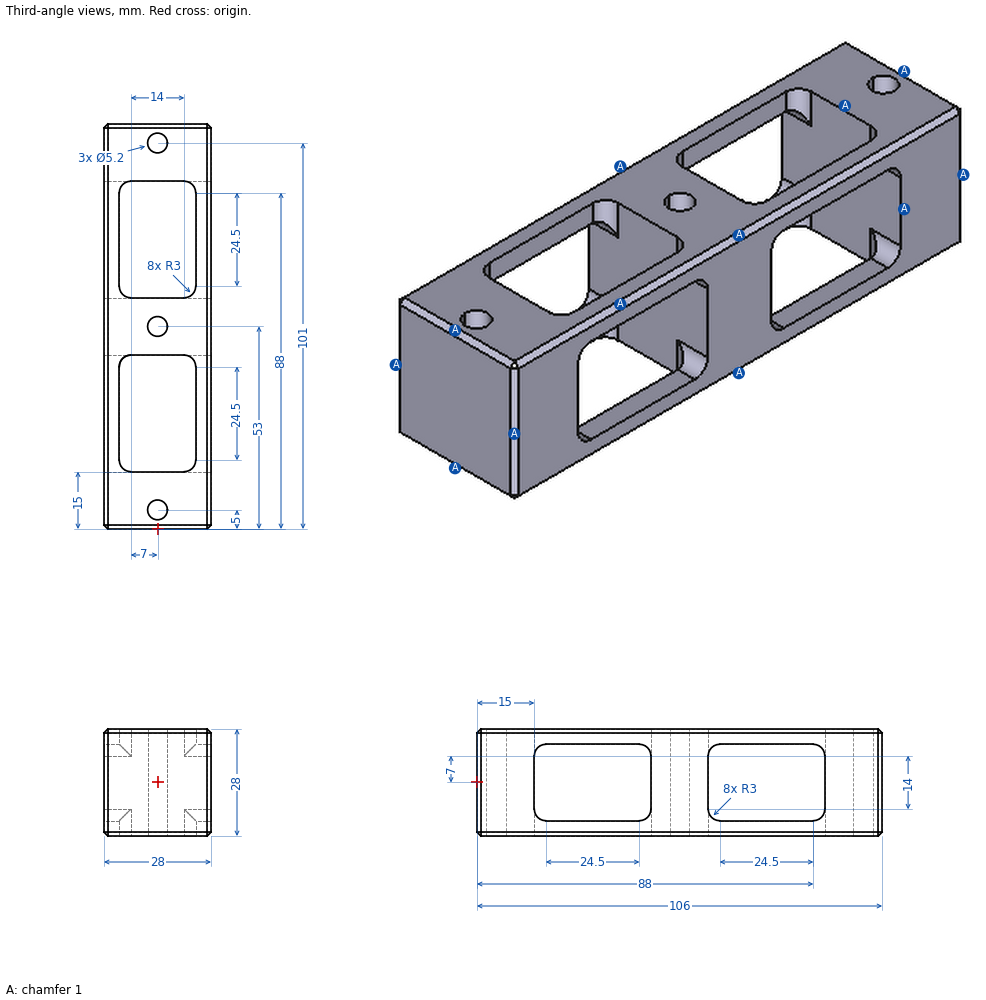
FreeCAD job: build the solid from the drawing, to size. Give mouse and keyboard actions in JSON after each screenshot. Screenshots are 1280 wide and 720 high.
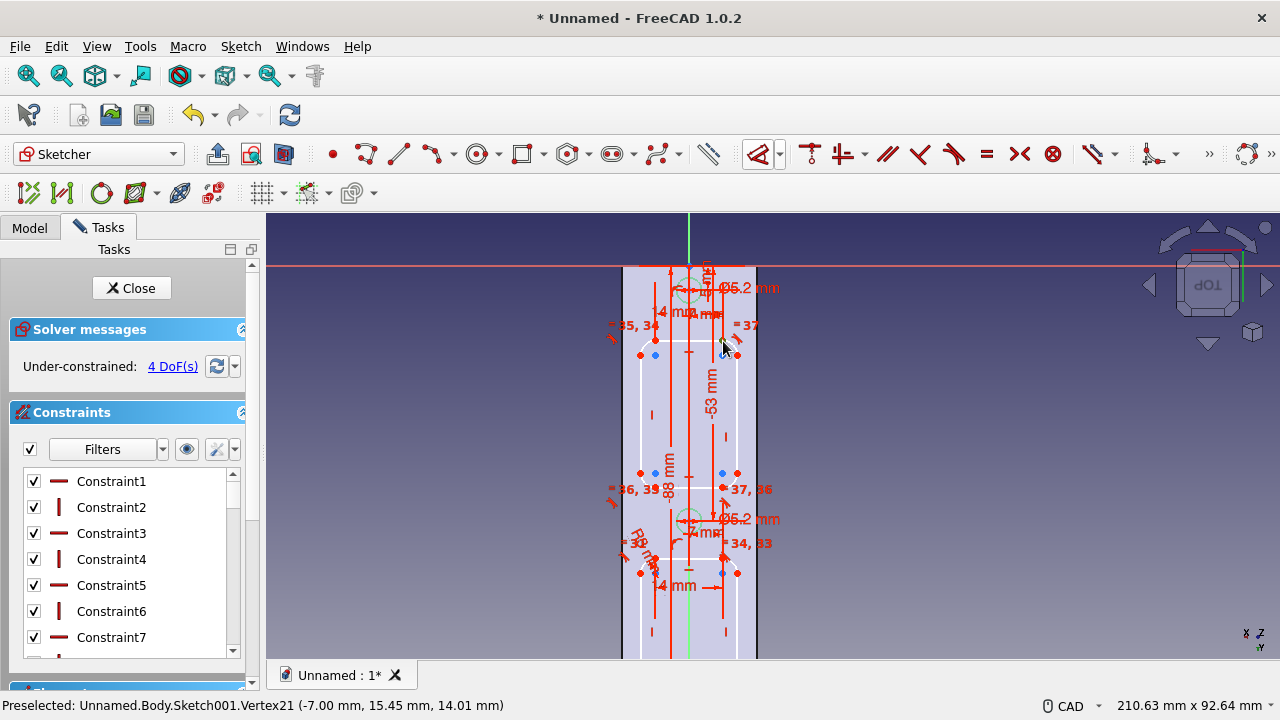
{"action": "key", "text": "i"}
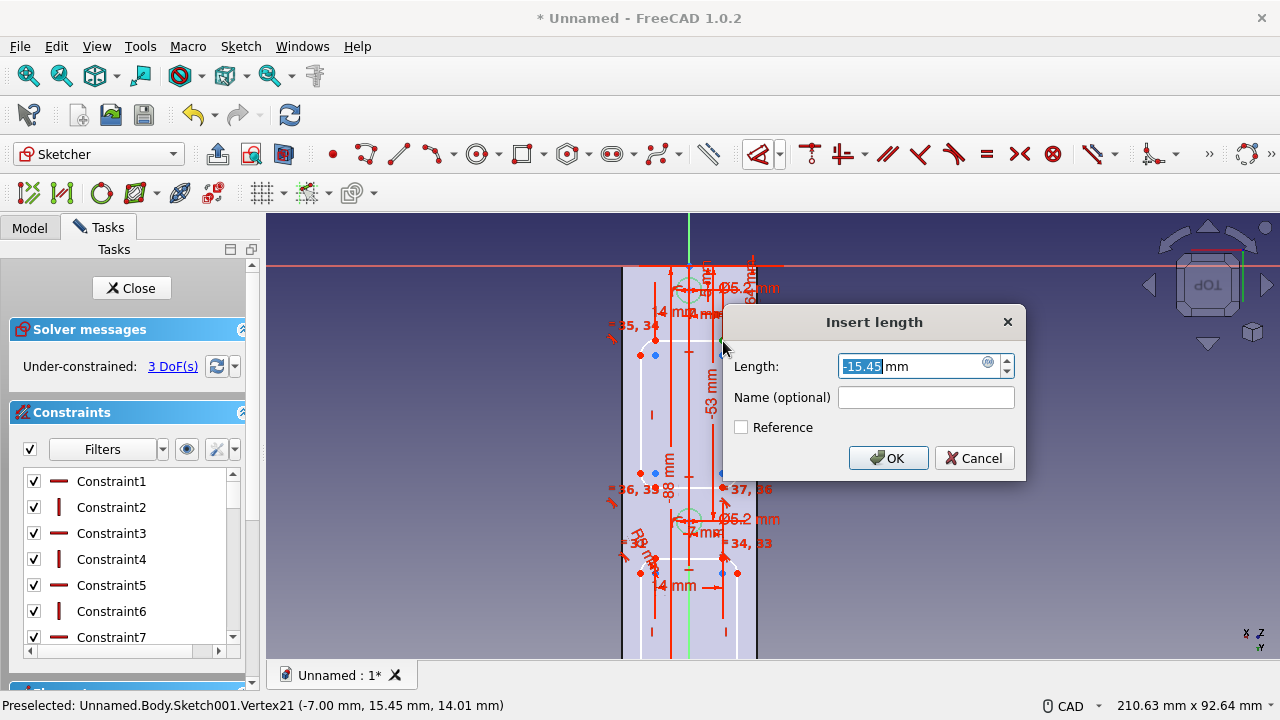
{"action": "type", "text": "-15"}
{"action": "key", "text": "Return"}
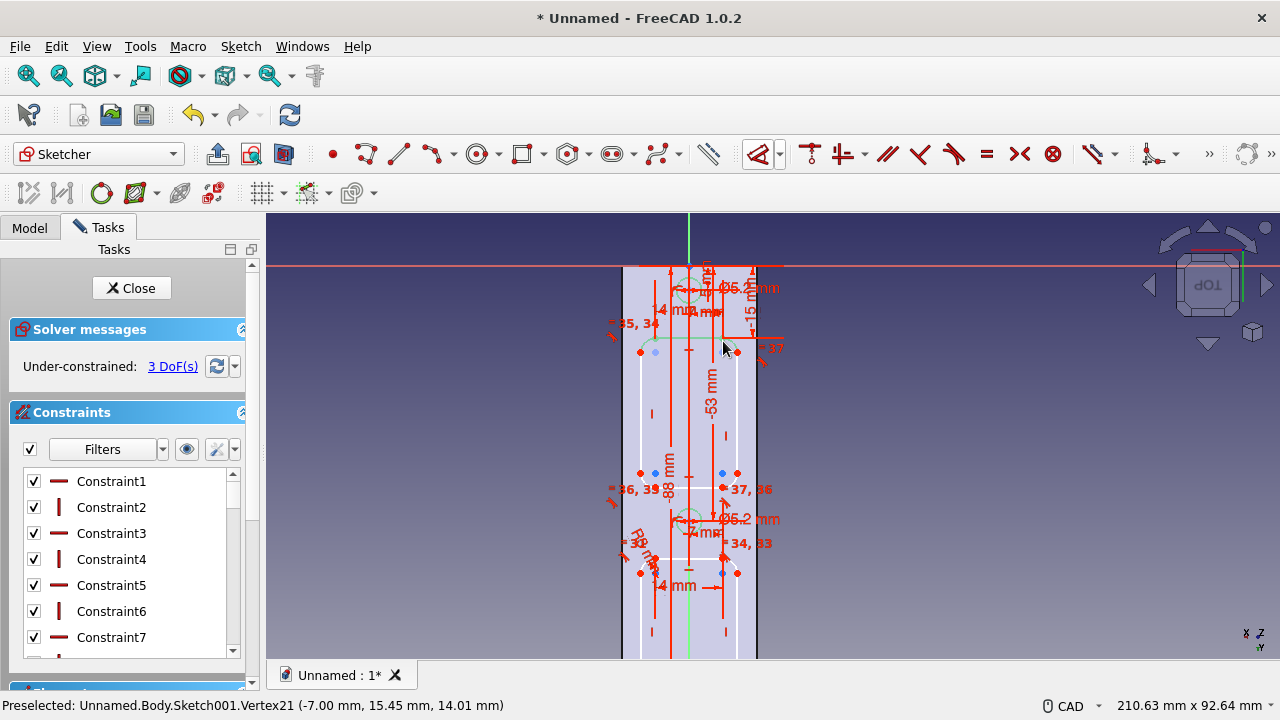
{"action": "scroll", "coordinate": [723, 339], "scroll_direction": "down", "scroll_amount": 3}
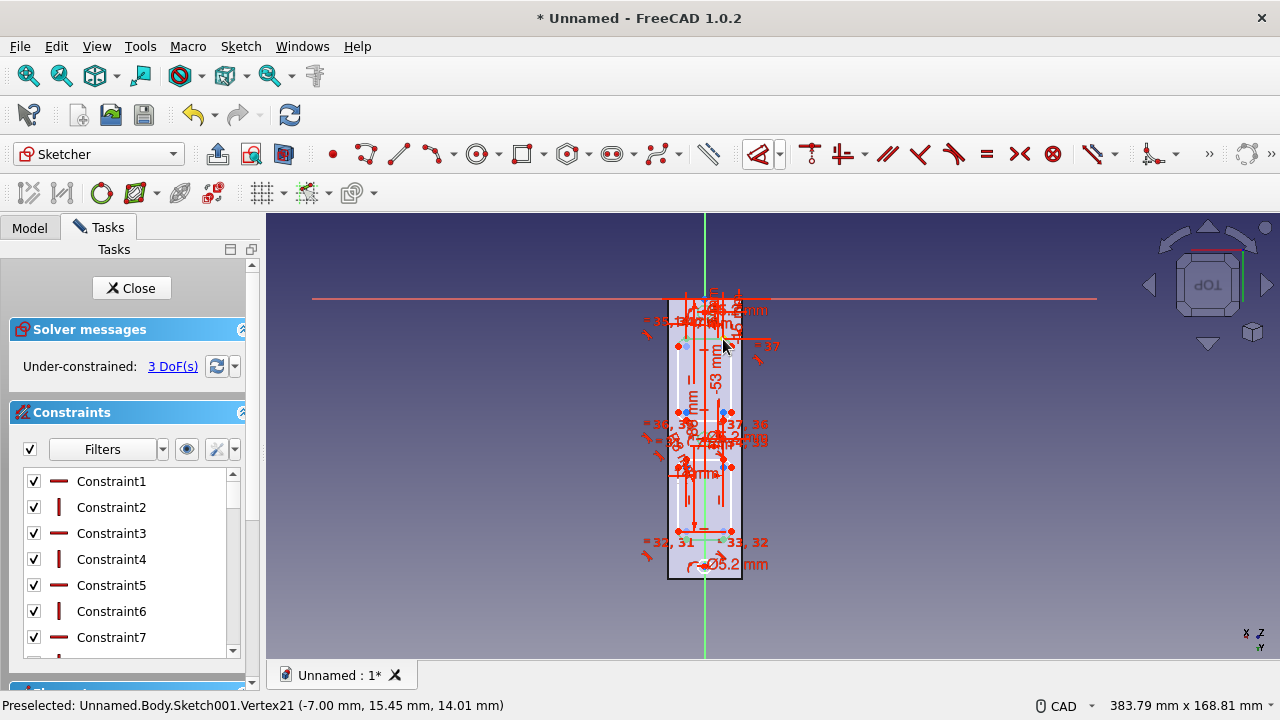
{"action": "left_click", "coordinate": [705, 566]}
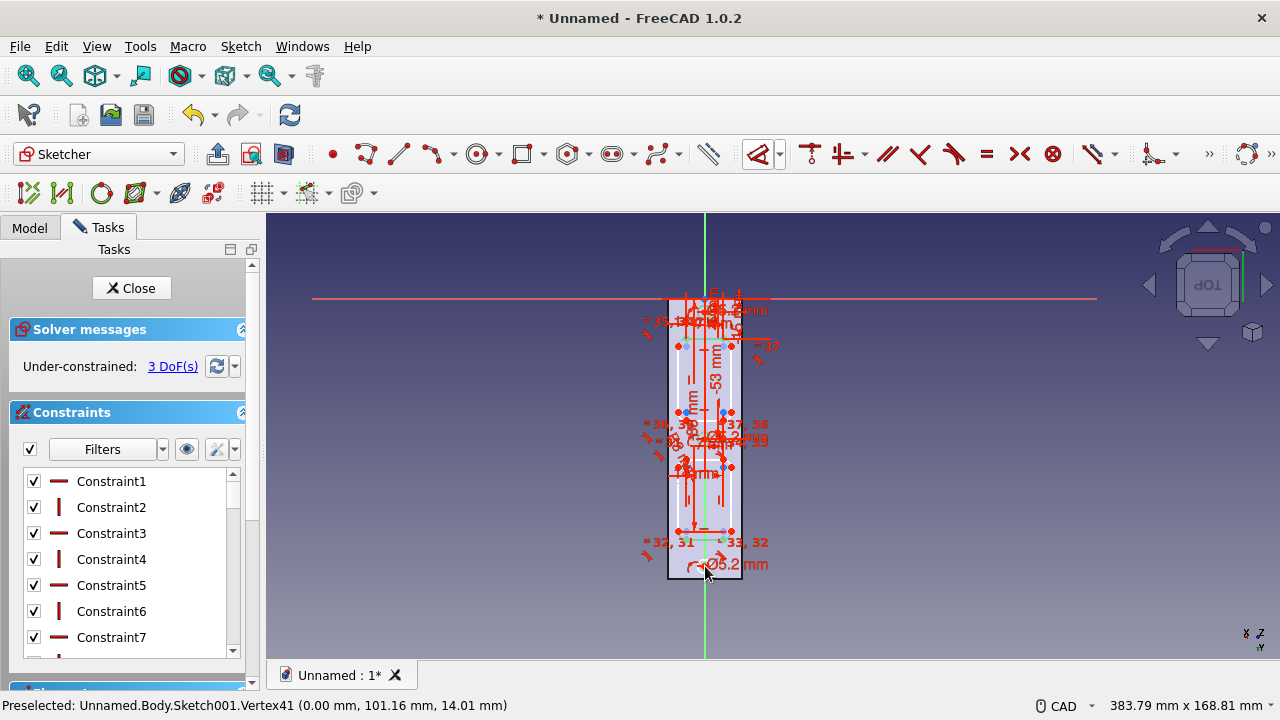
{"action": "left_click", "coordinate": [780, 154]}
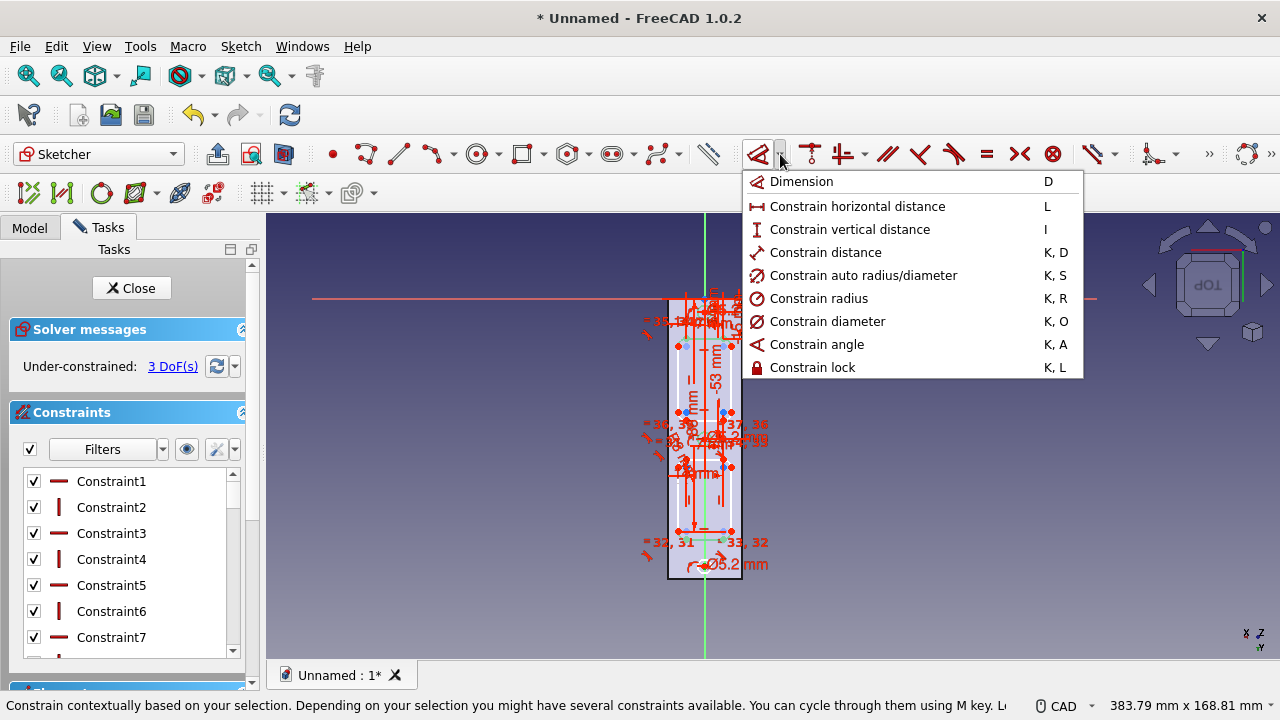
{"action": "left_click", "coordinate": [913, 230]}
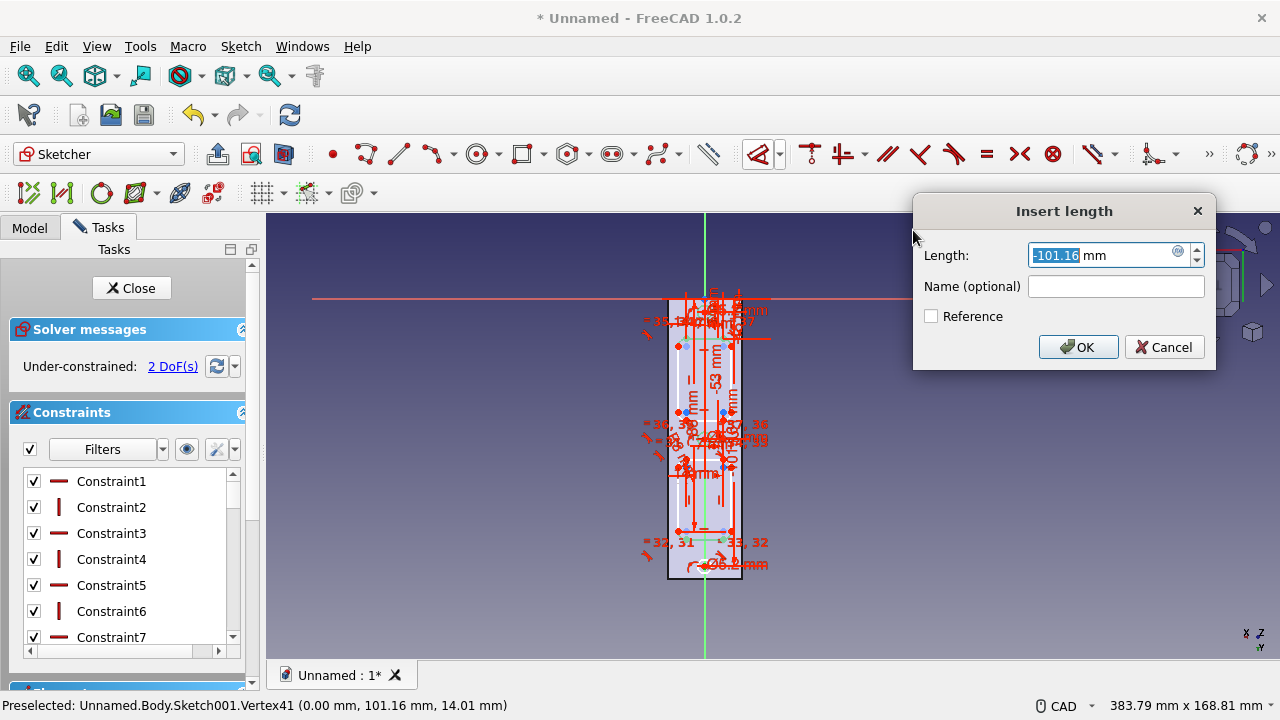
{"action": "type", "text": "-101"}
{"action": "key", "text": "Return"}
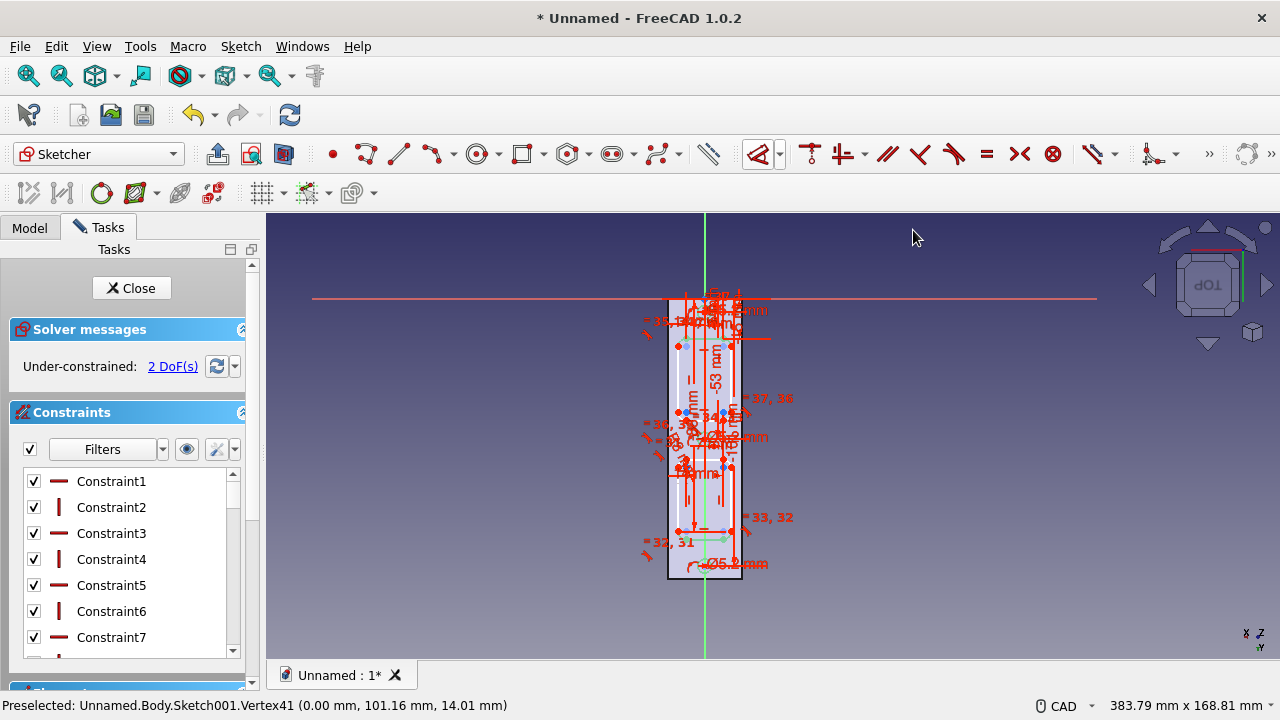
{"action": "left_click", "coordinate": [678, 487]}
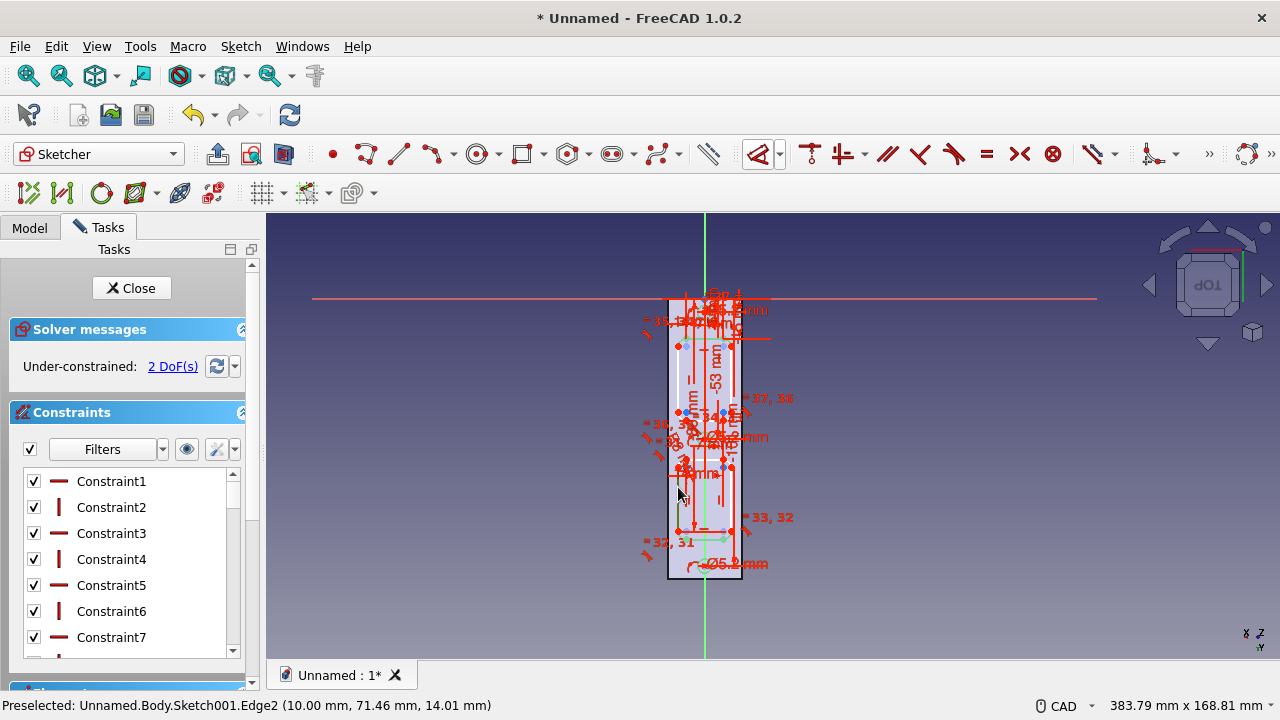
{"action": "left_click", "coordinate": [780, 154]}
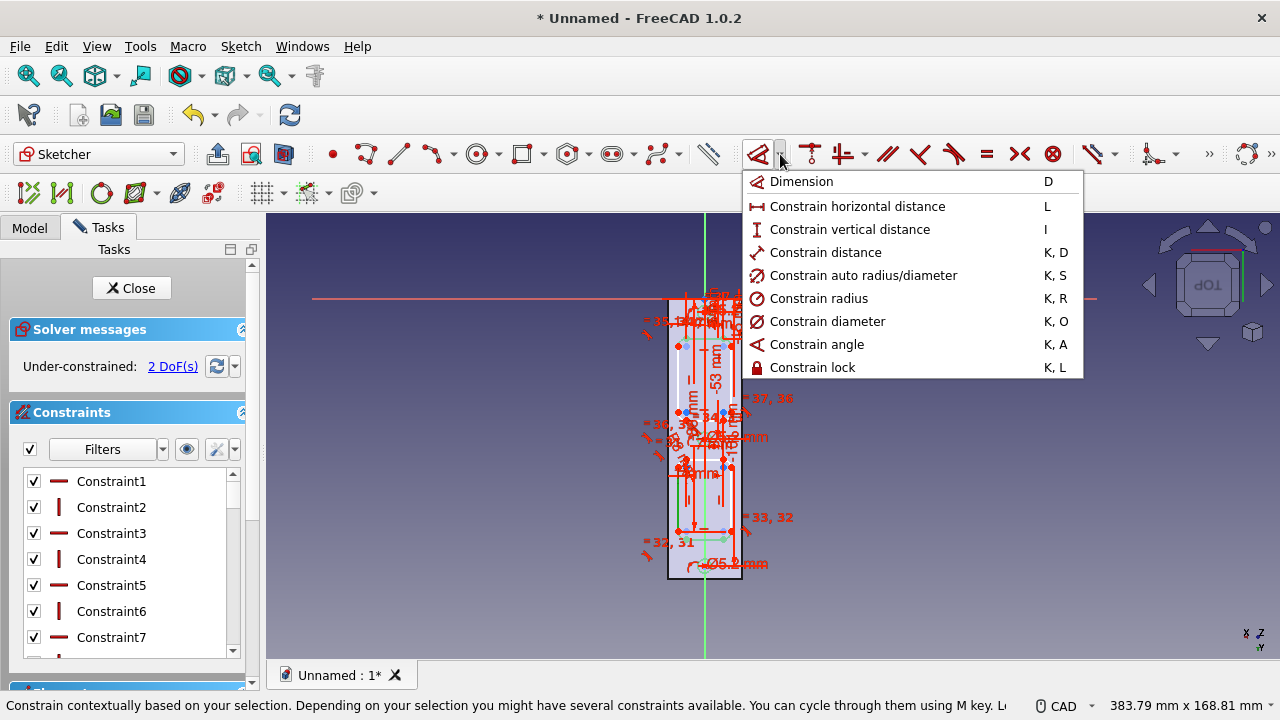
{"action": "left_click", "coordinate": [913, 230]}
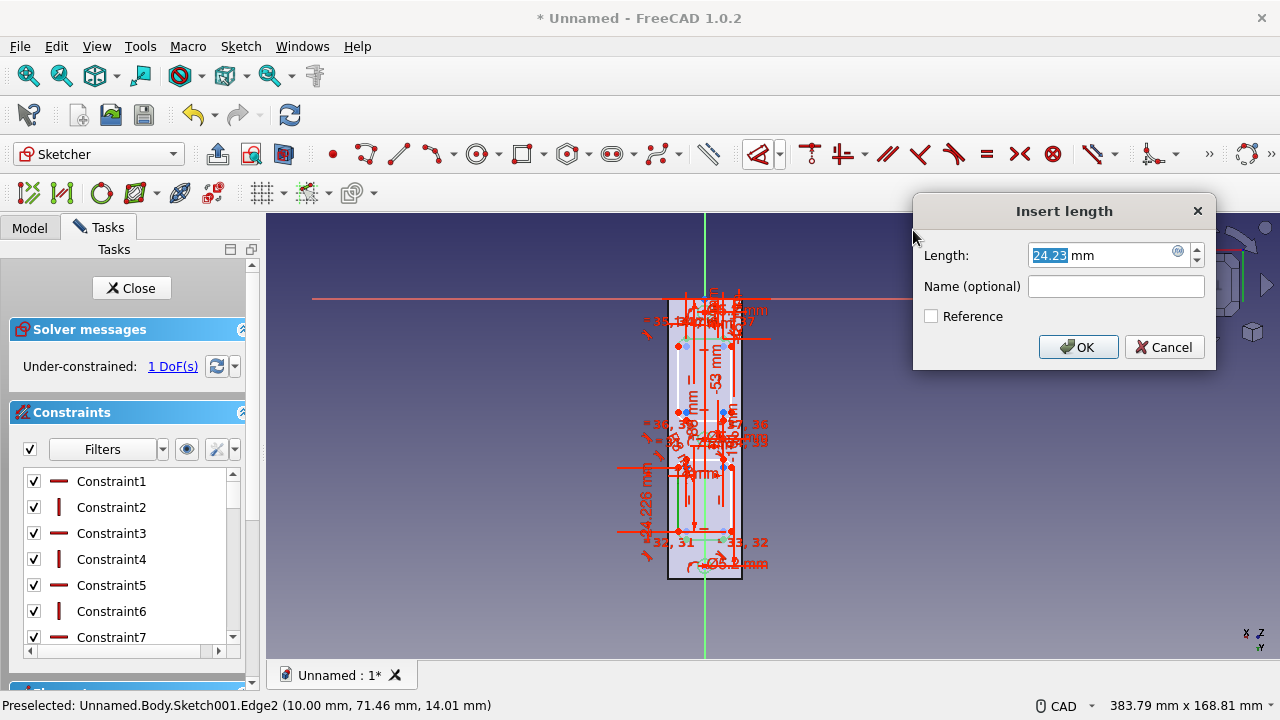
{"action": "type", "text": "24.5"}
{"action": "key", "text": "Return"}